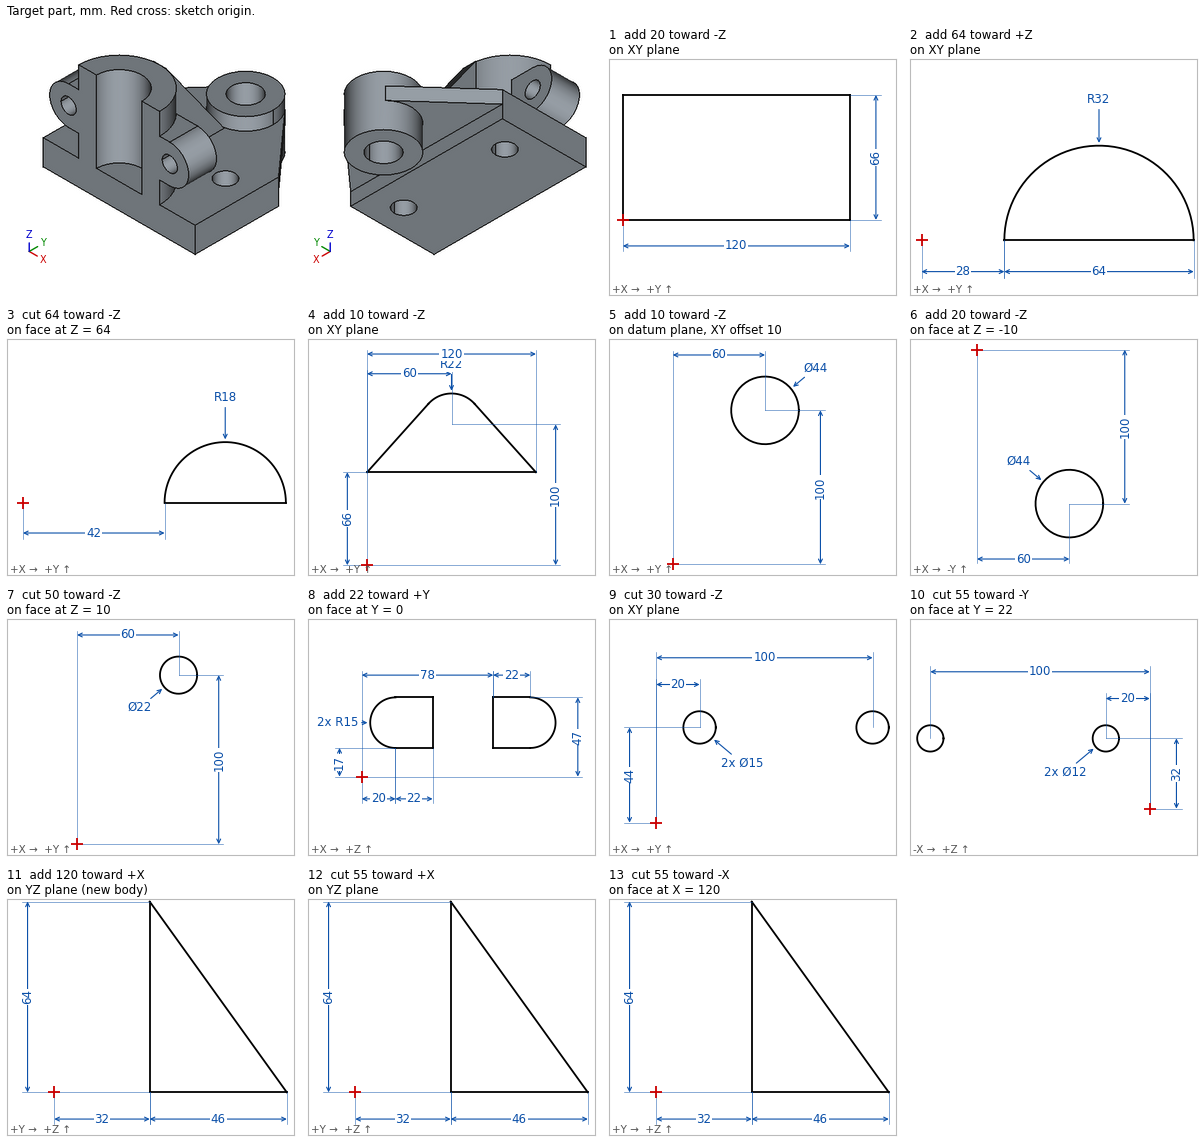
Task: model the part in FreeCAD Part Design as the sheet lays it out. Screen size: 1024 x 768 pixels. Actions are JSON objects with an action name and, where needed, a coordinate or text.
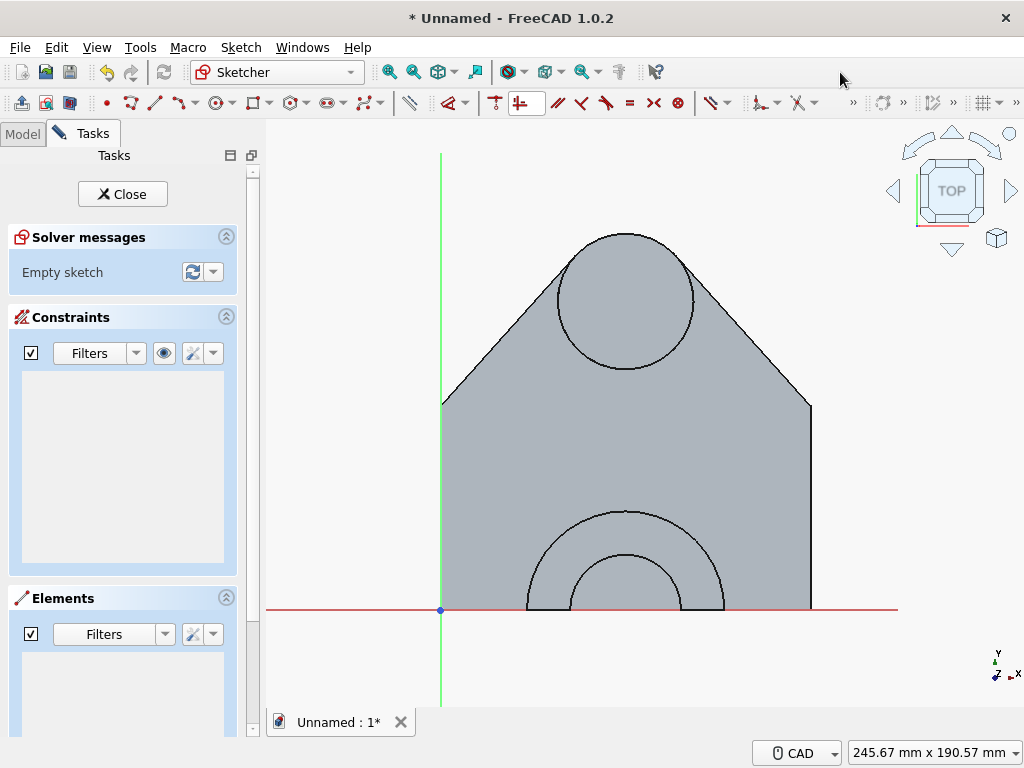
{"action": "left_click", "coordinate": [70, 104]}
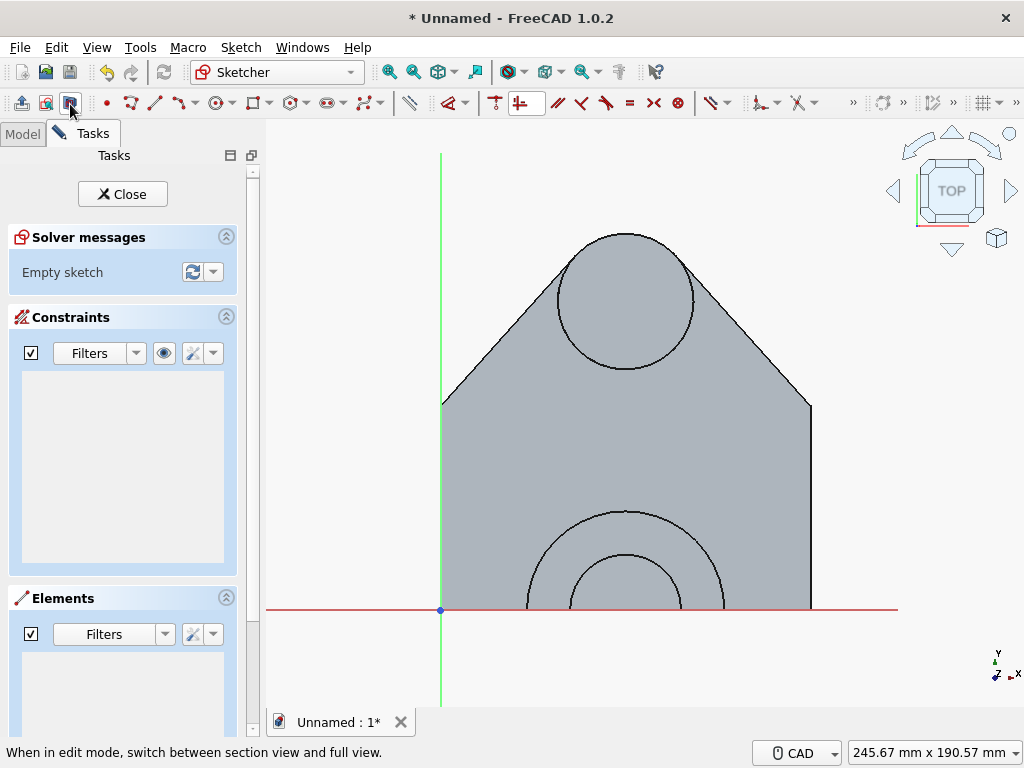
{"action": "scroll", "coordinate": [635, 279], "scroll_direction": "up", "scroll_amount": 9}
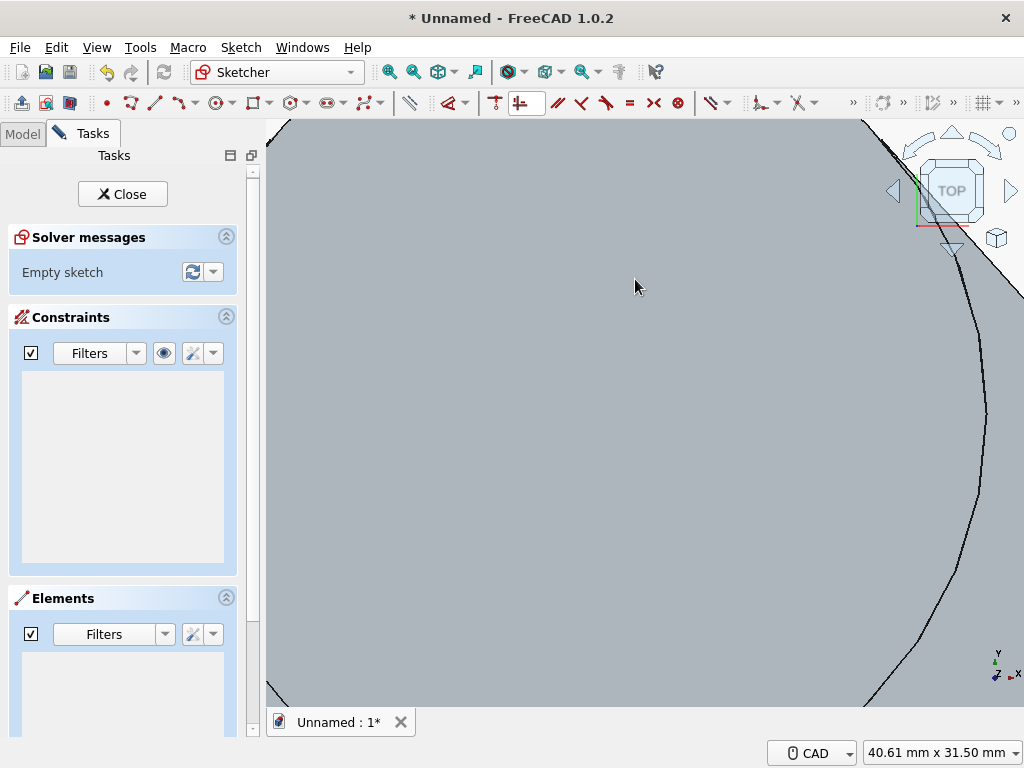
{"action": "left_click", "coordinate": [216, 104]}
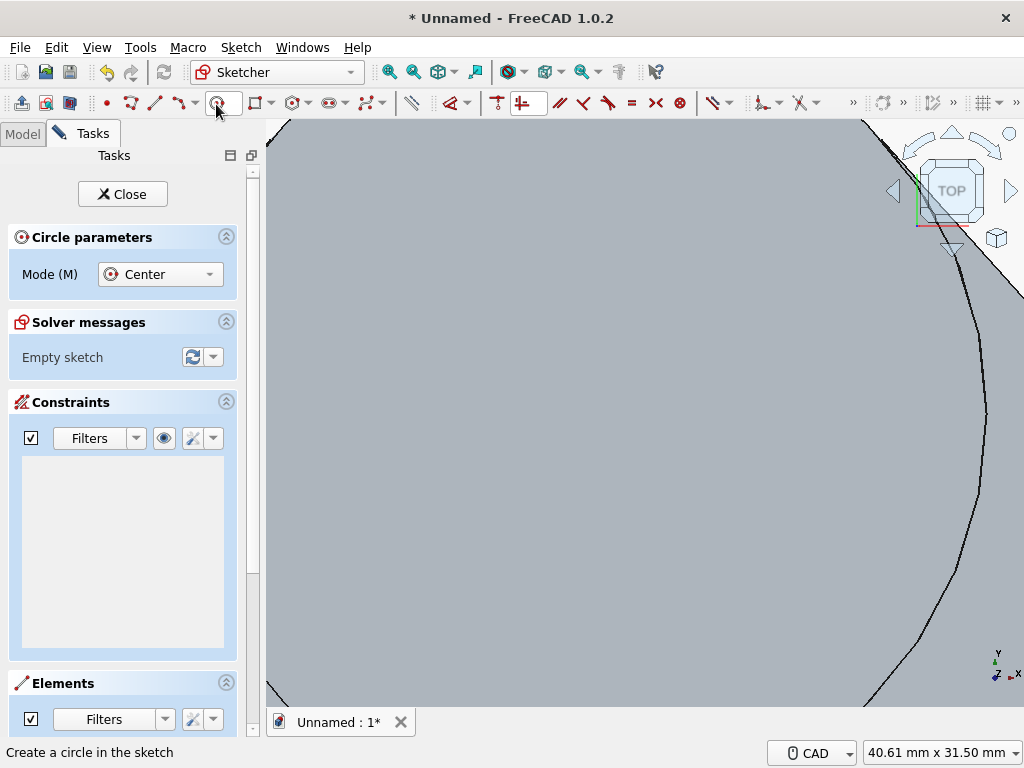
{"action": "left_click", "coordinate": [576, 414]}
{"action": "left_click", "coordinate": [721, 269]}
{"action": "key", "text": "Escape"}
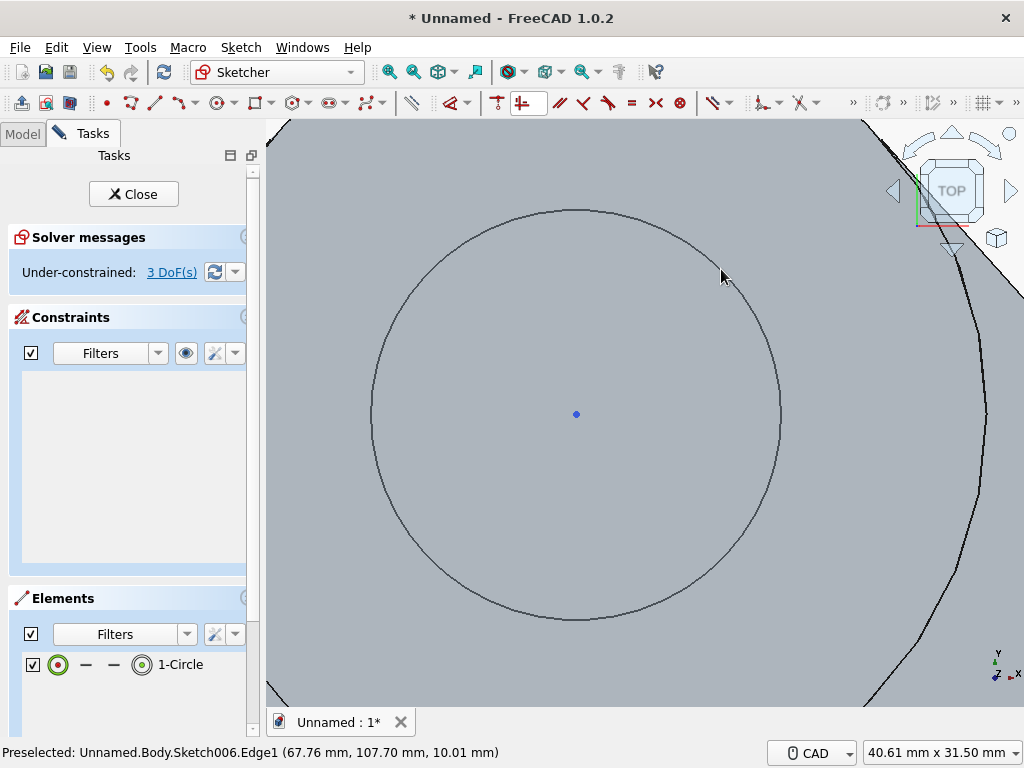
{"action": "left_click", "coordinate": [450, 104]}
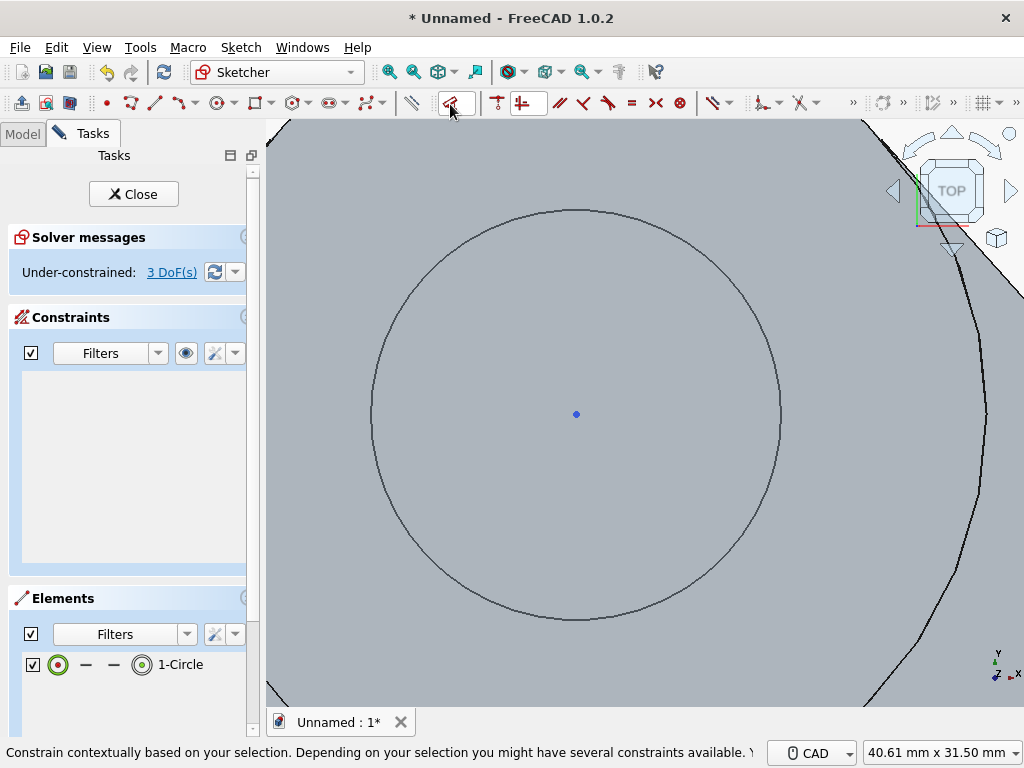
{"action": "left_click", "coordinate": [721, 270]}
{"action": "left_click", "coordinate": [744, 247]}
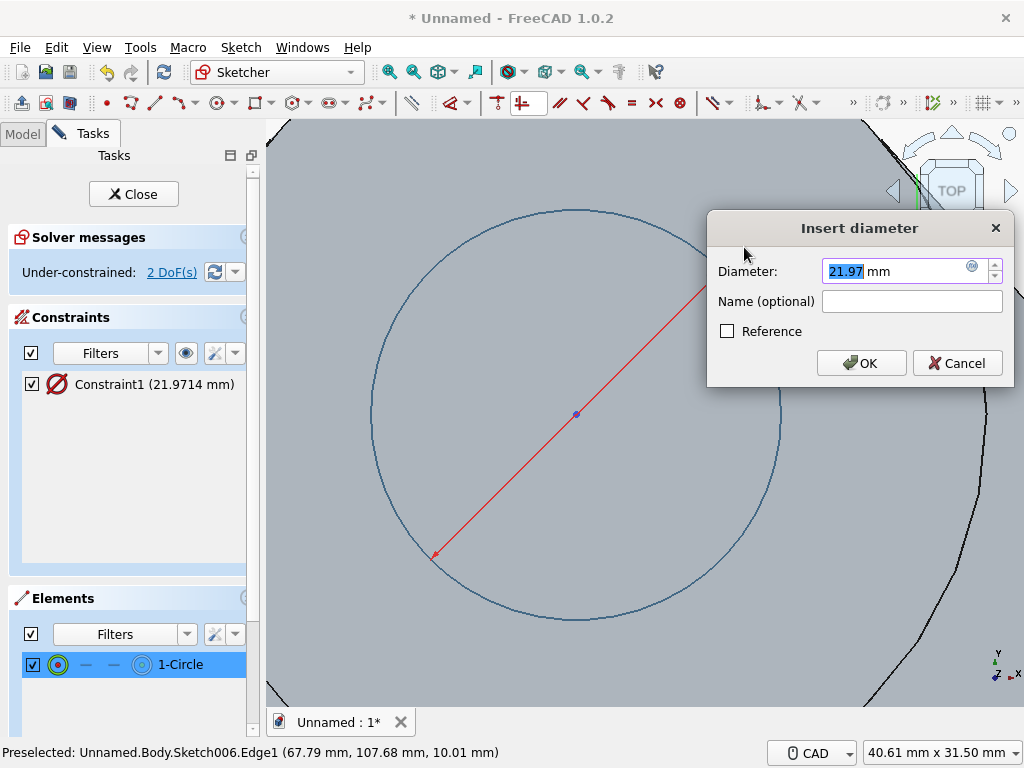
{"action": "type", "text": "22"}
{"action": "key", "text": "Return"}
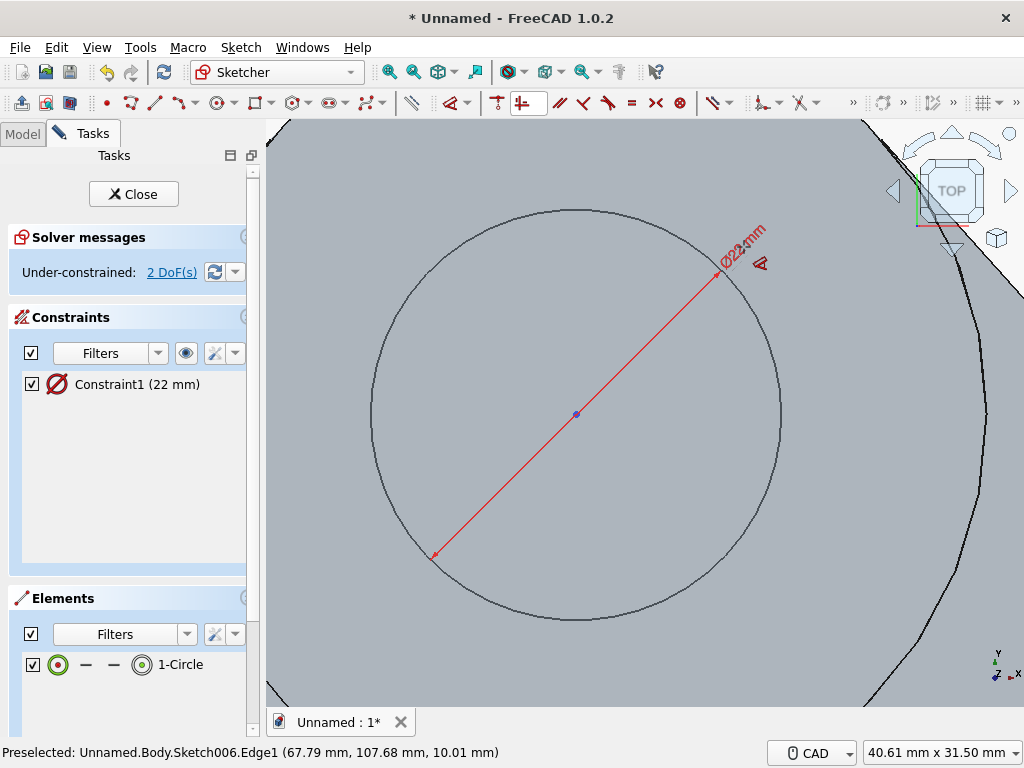
{"action": "left_click", "coordinate": [576, 415]}
{"action": "left_click", "coordinate": [435, 381]}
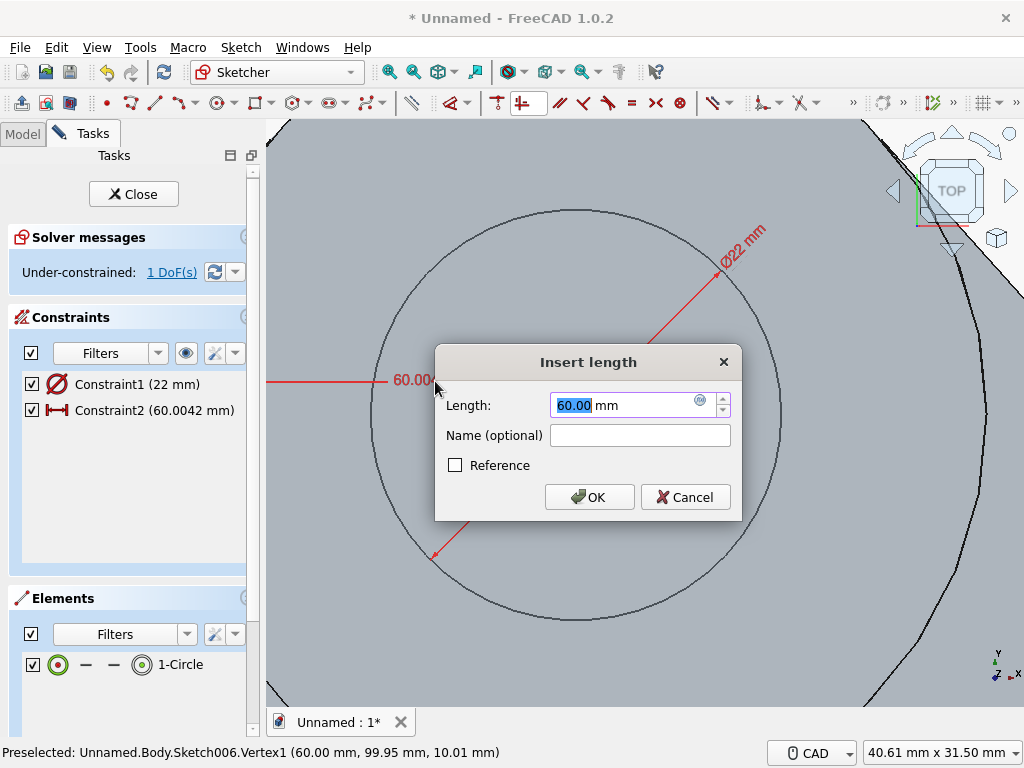
{"action": "type", "text": "60"}
{"action": "key", "text": "Return"}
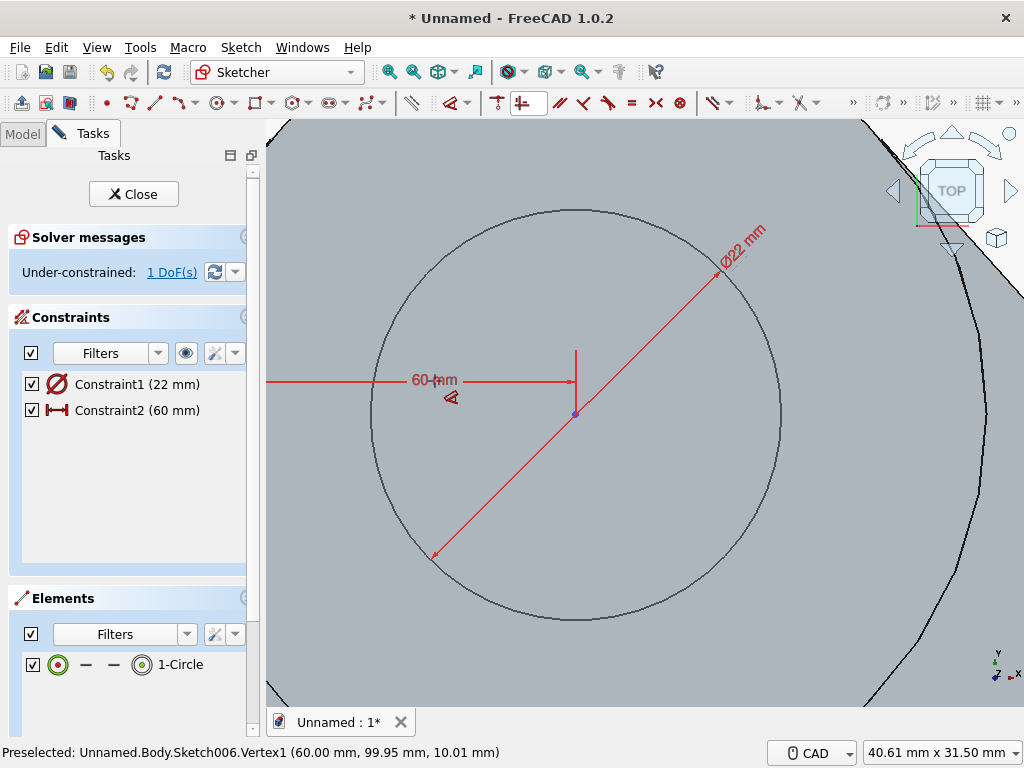
{"action": "left_click", "coordinate": [576, 415]}
{"action": "left_click", "coordinate": [610, 547]}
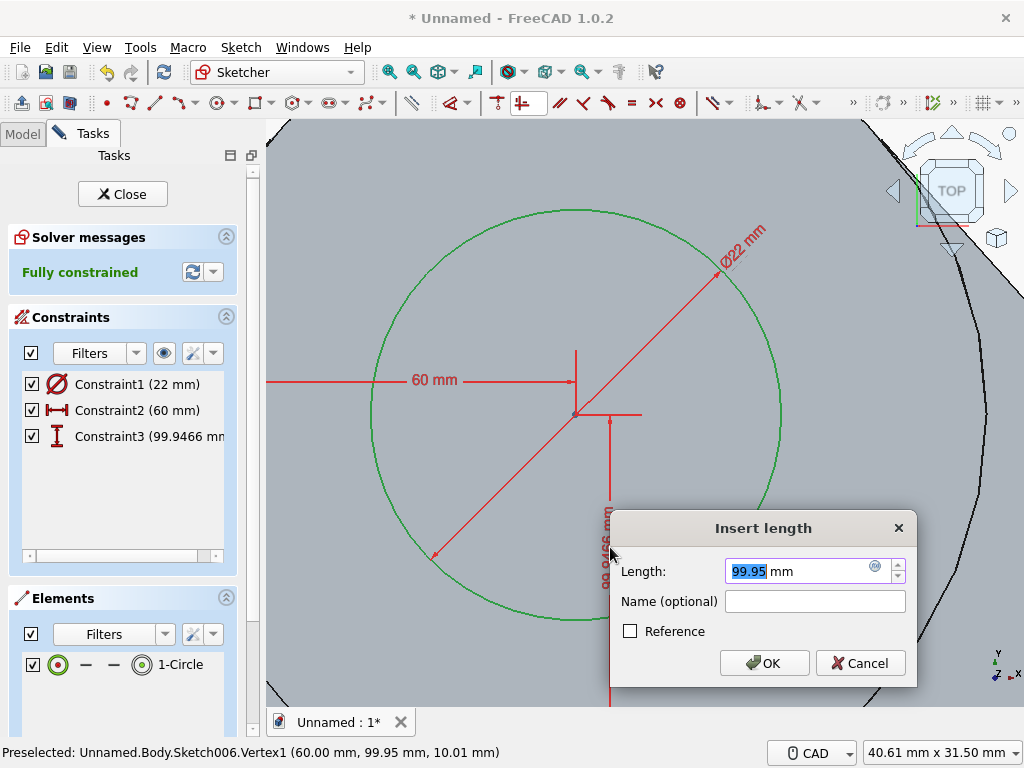
{"action": "type", "text": "100"}
{"action": "key", "text": "Return"}
{"action": "key", "text": "Escape"}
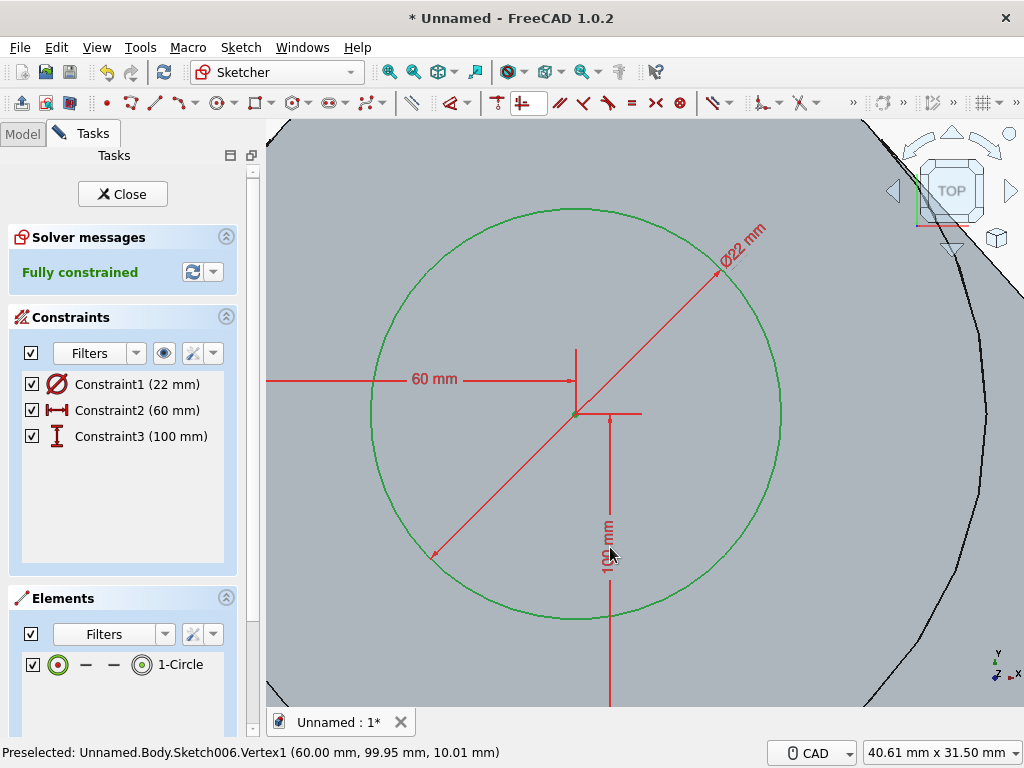
{"action": "left_click", "coordinate": [123, 194]}